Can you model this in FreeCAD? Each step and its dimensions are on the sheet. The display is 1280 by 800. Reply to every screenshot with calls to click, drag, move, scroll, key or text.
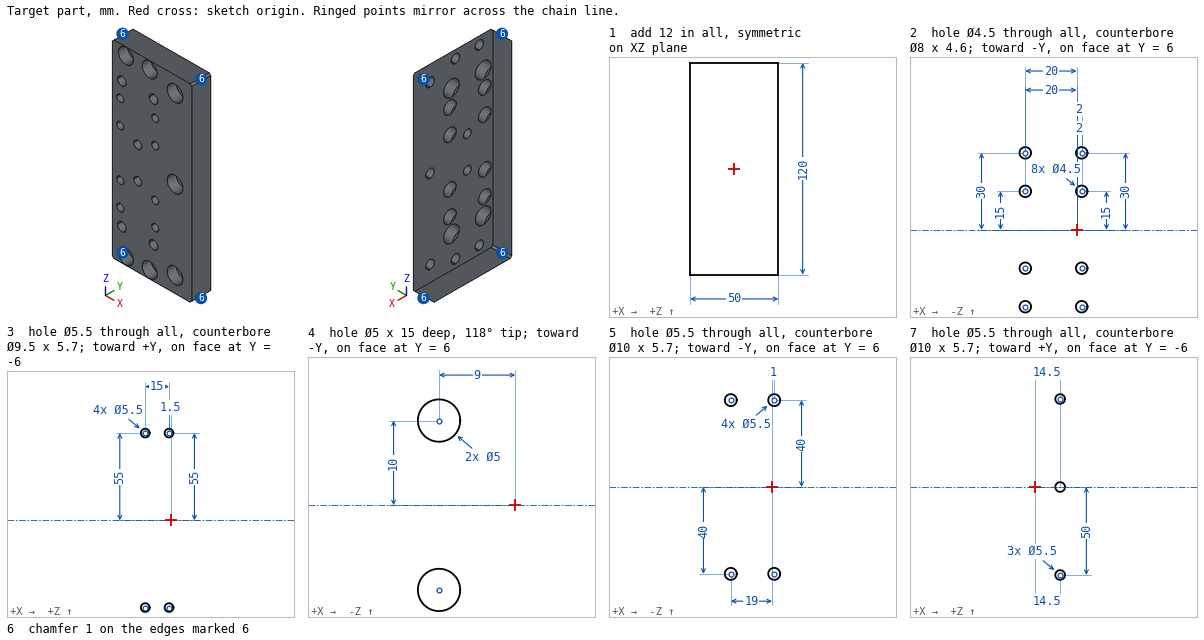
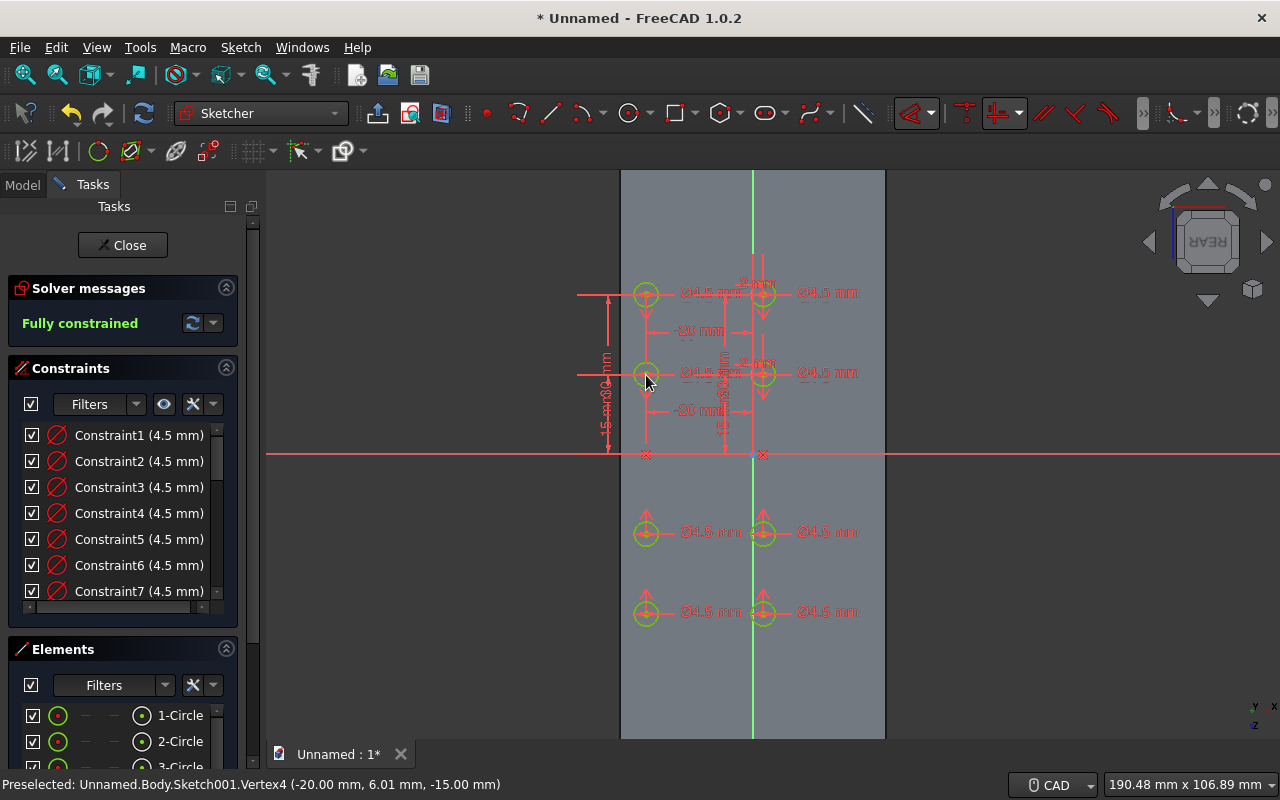
click(123, 245)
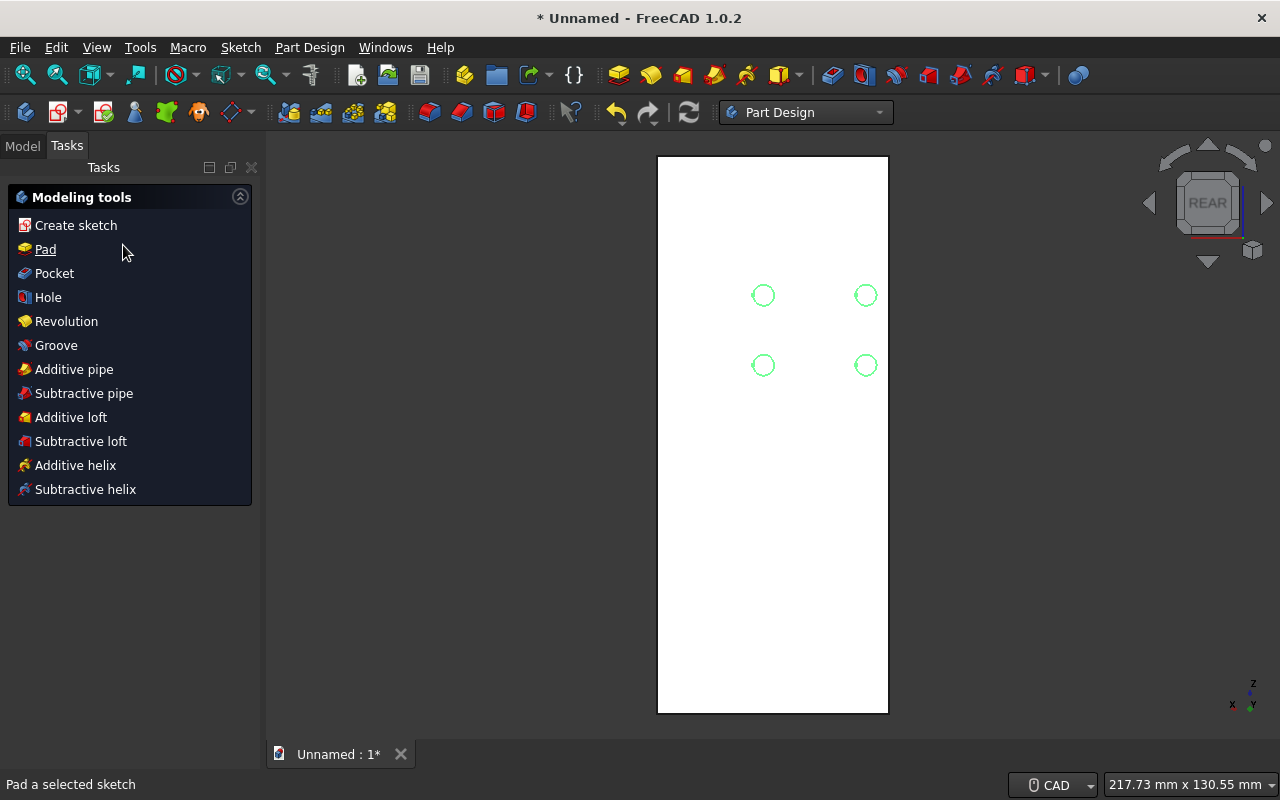
click(866, 76)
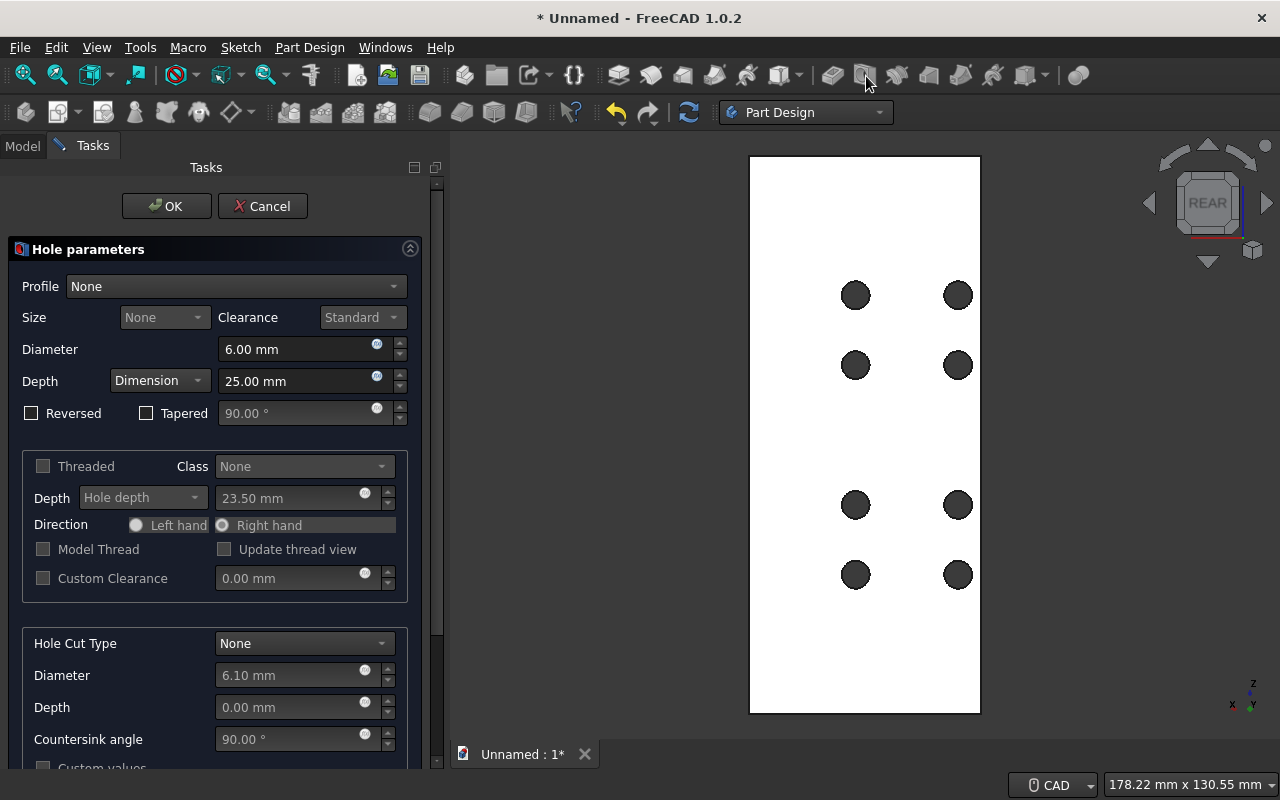
triple_click(305, 349)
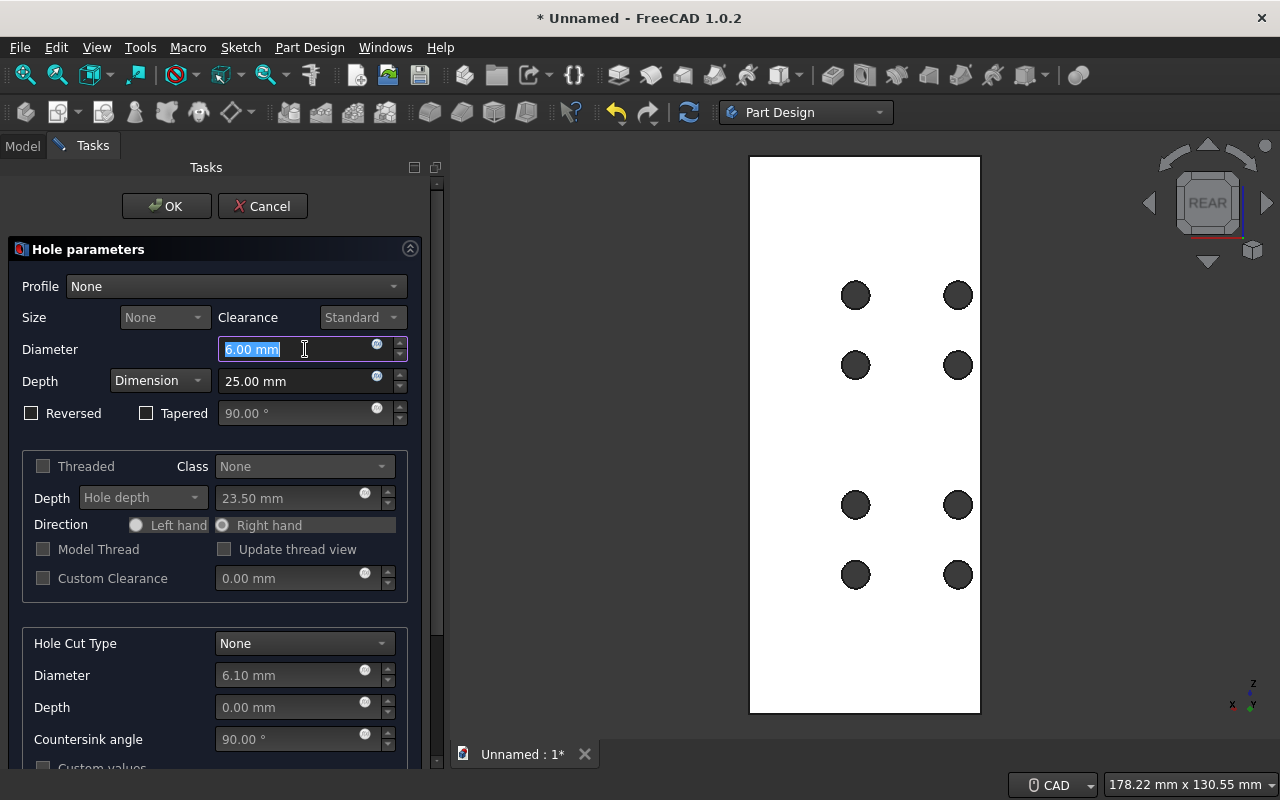
text(4.5)
key(Tab)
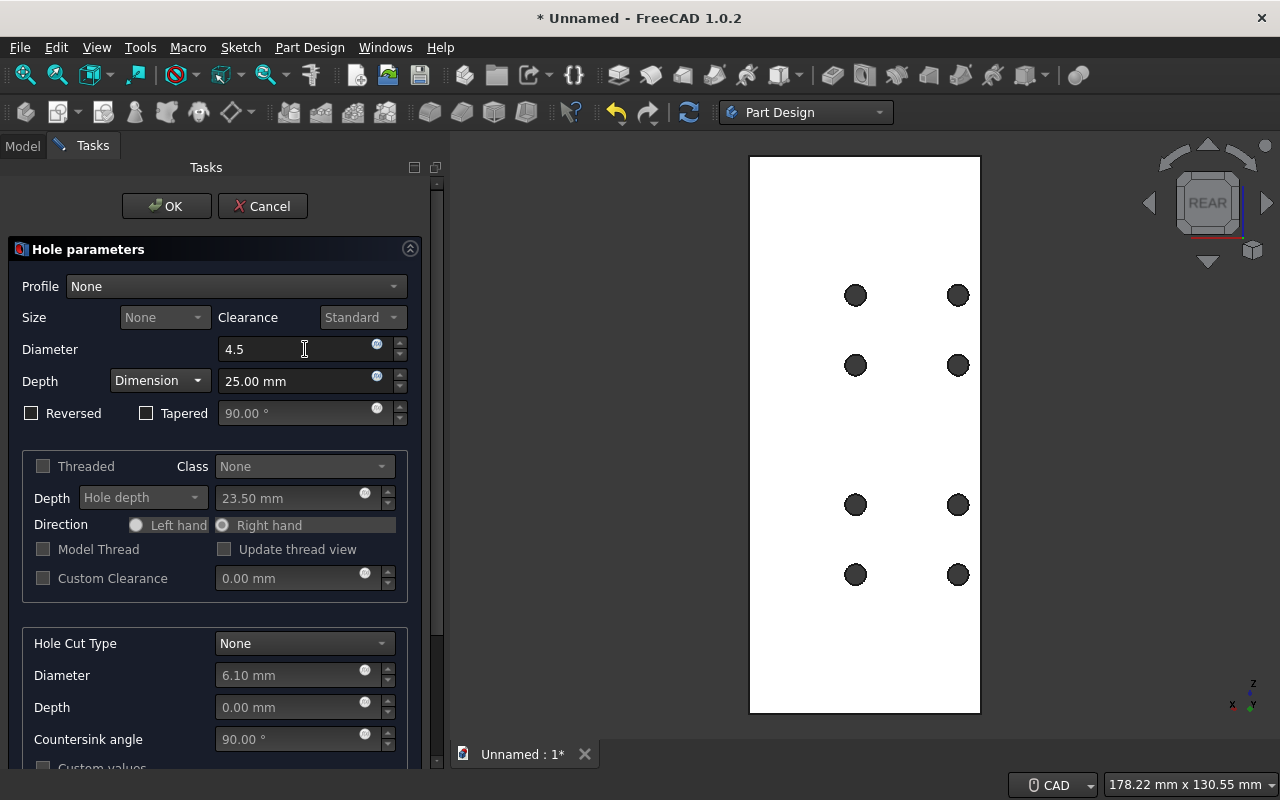
click(161, 380)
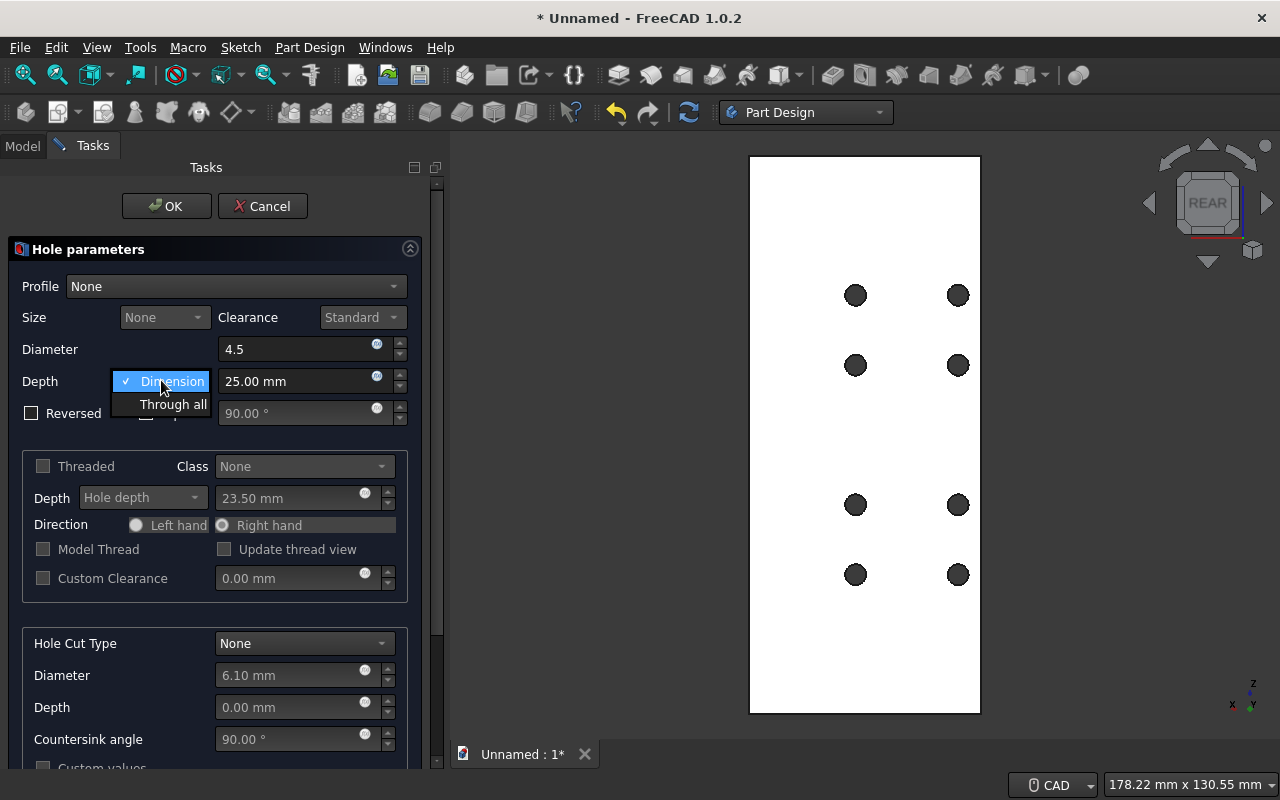
click(160, 404)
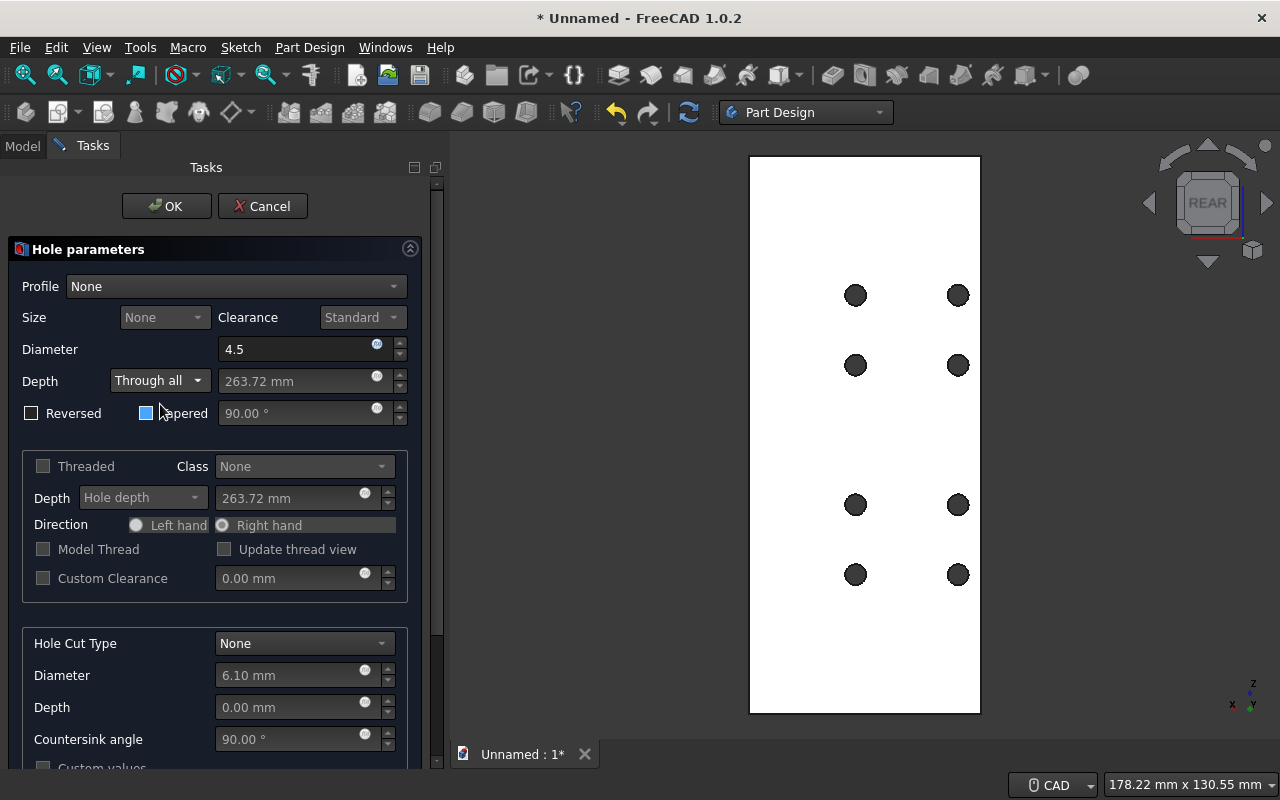
click(306, 644)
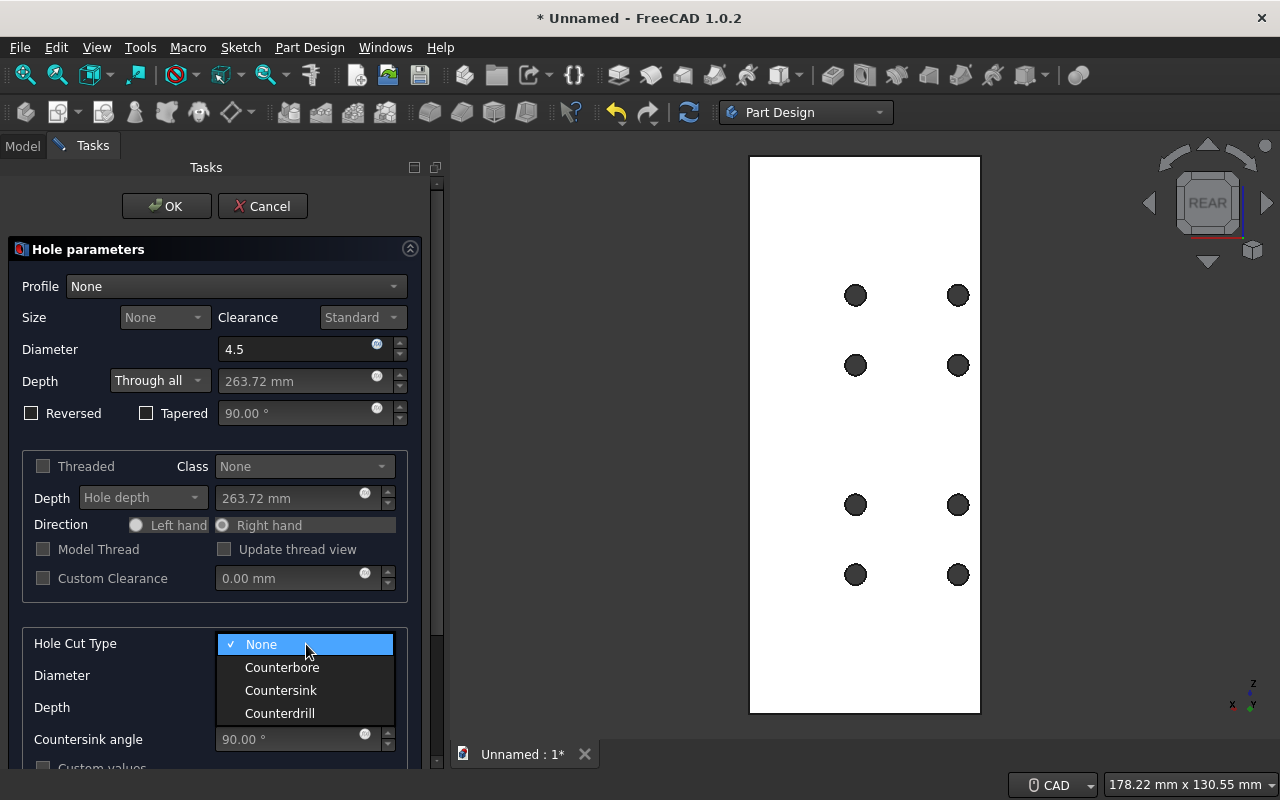
click(304, 668)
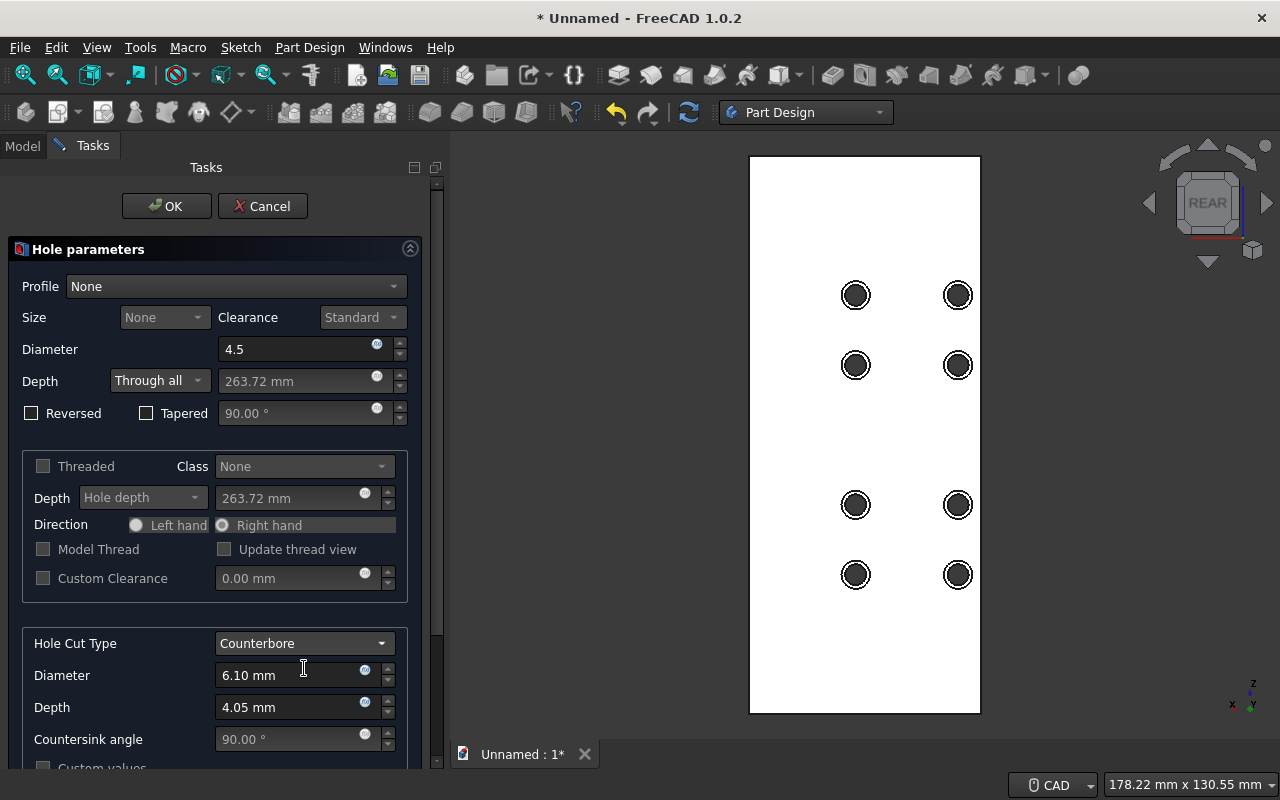
triple_click(298, 675)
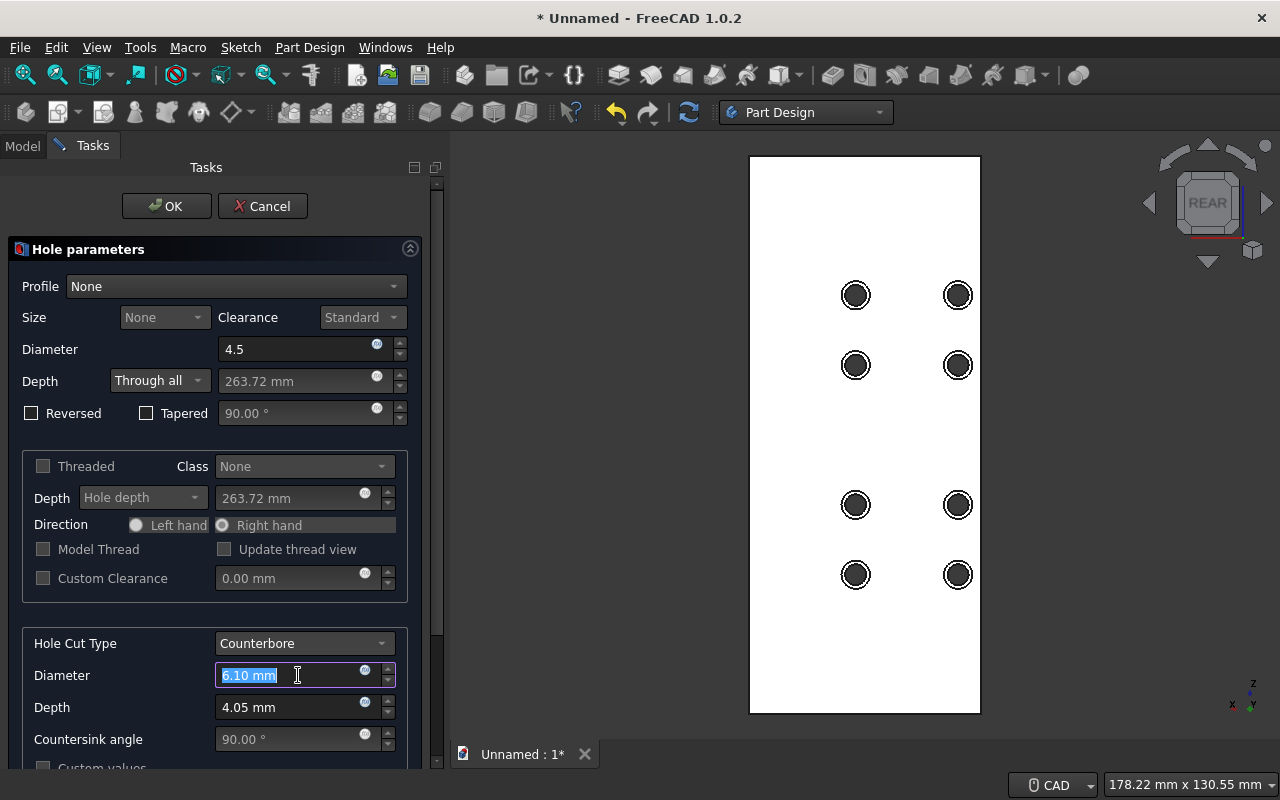
text(8)
key(Tab)